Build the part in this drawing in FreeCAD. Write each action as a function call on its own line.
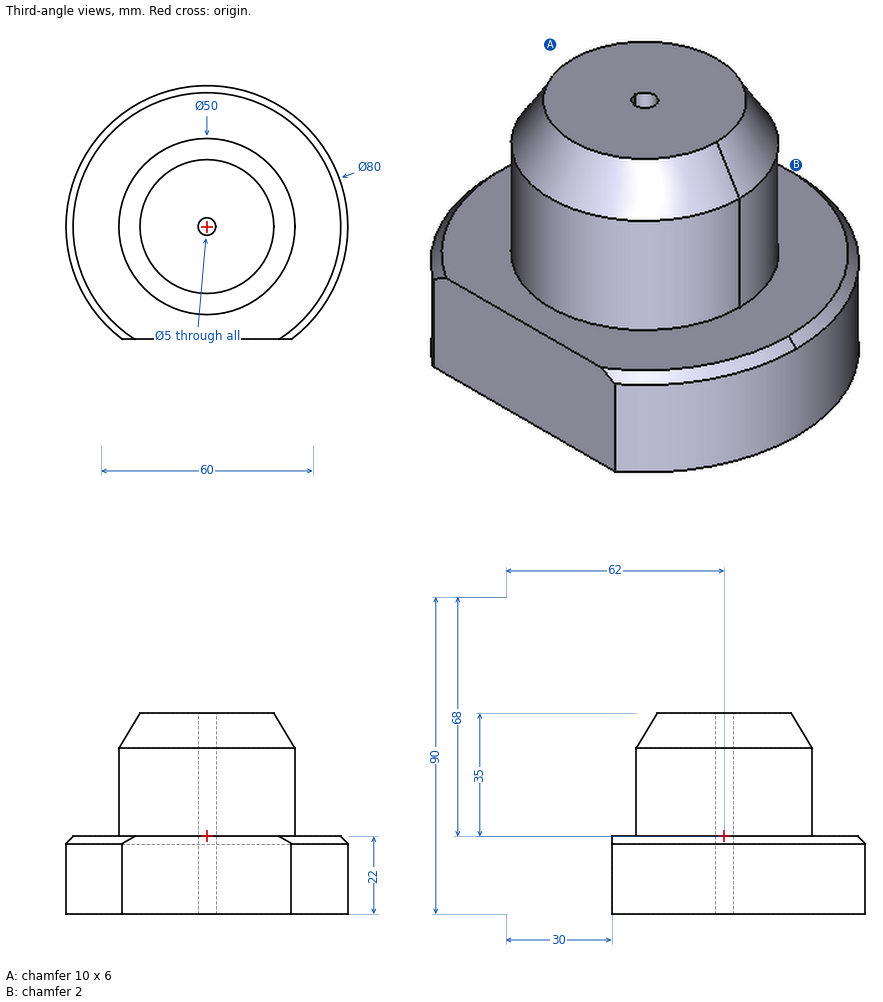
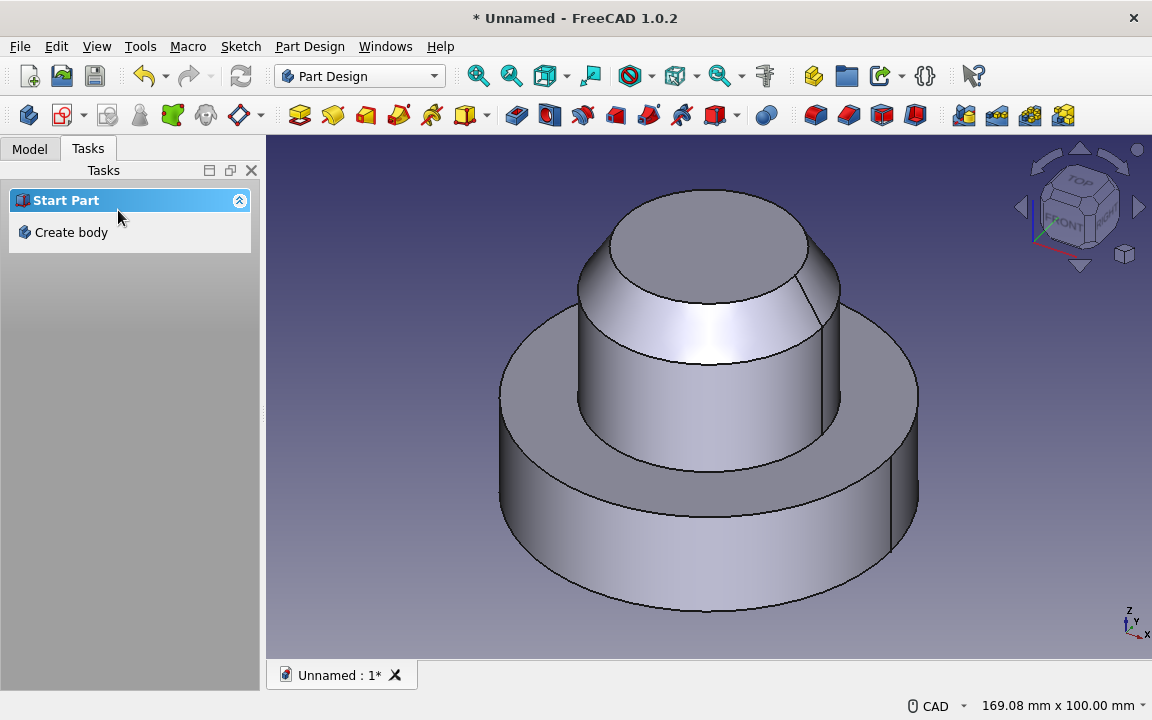
click(479, 76)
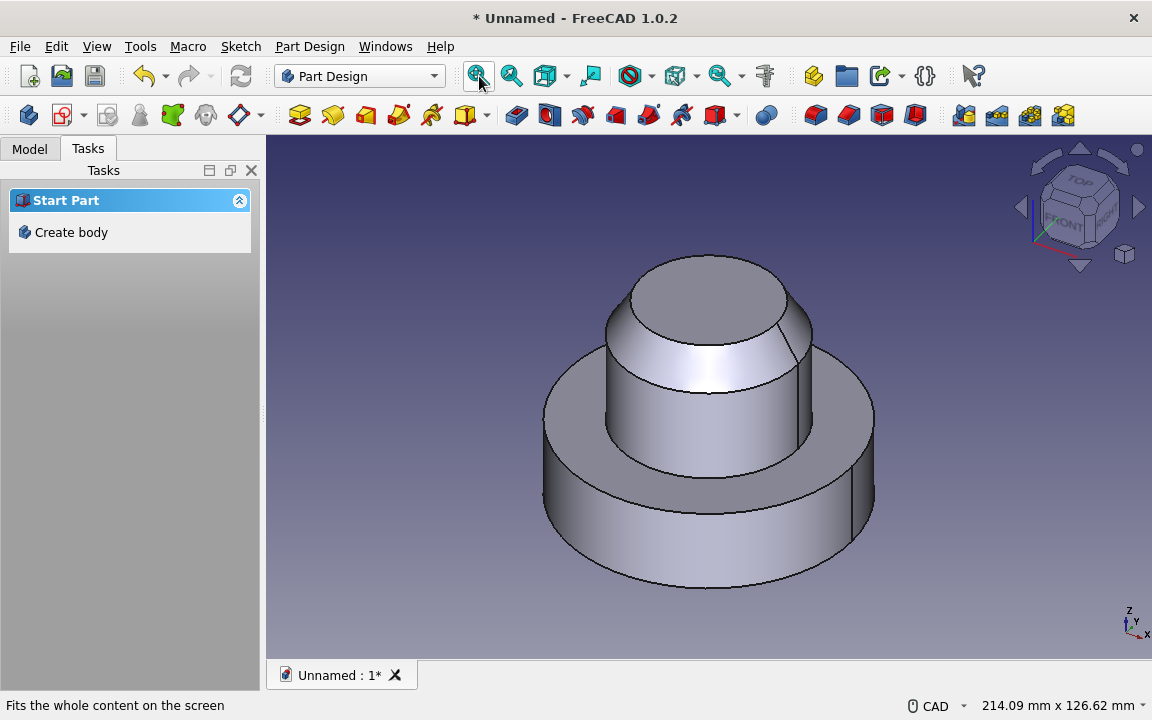
click(62, 116)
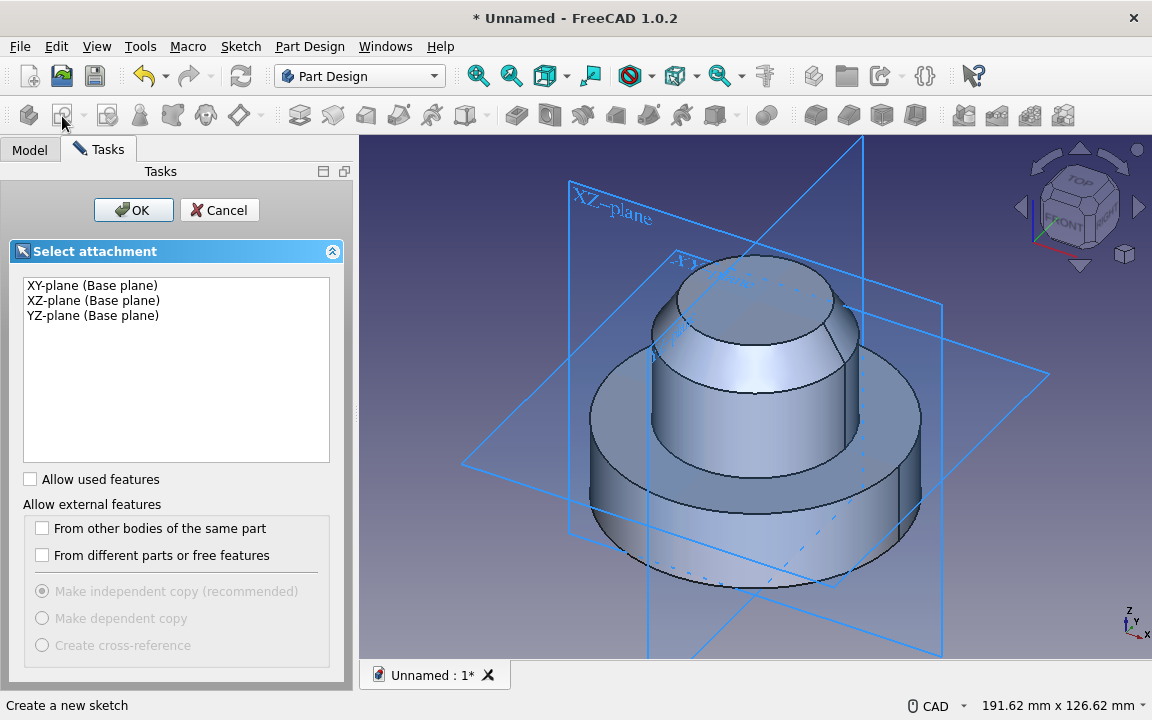
click(84, 316)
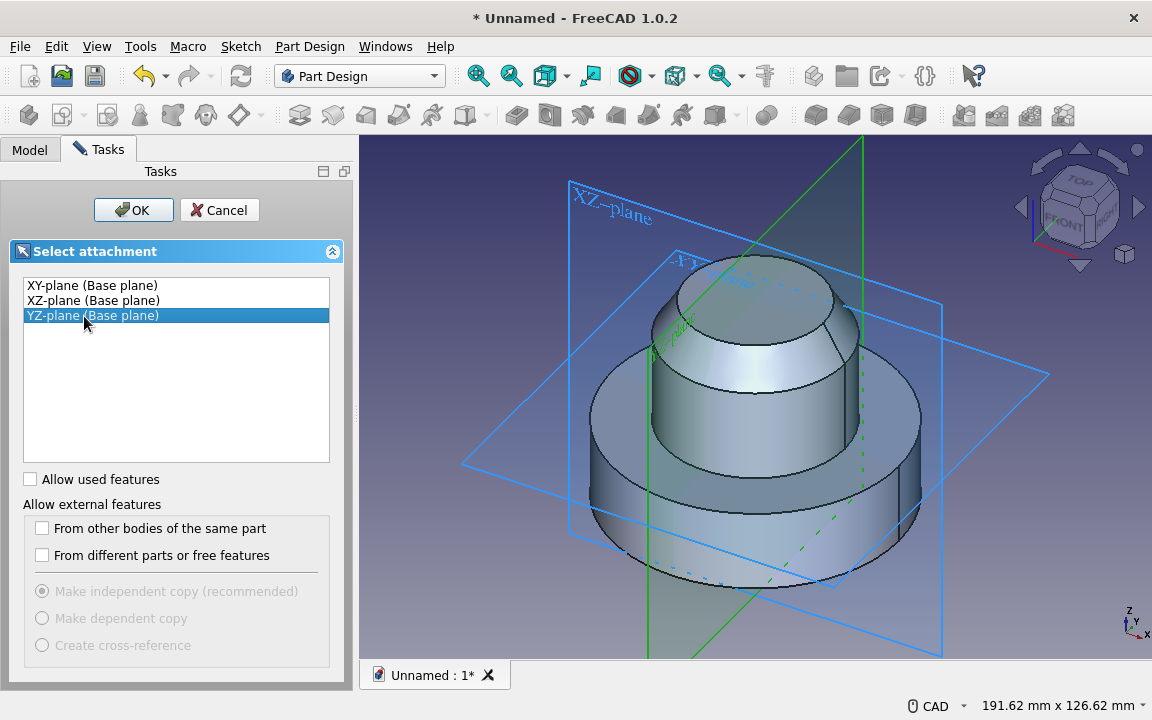
click(134, 210)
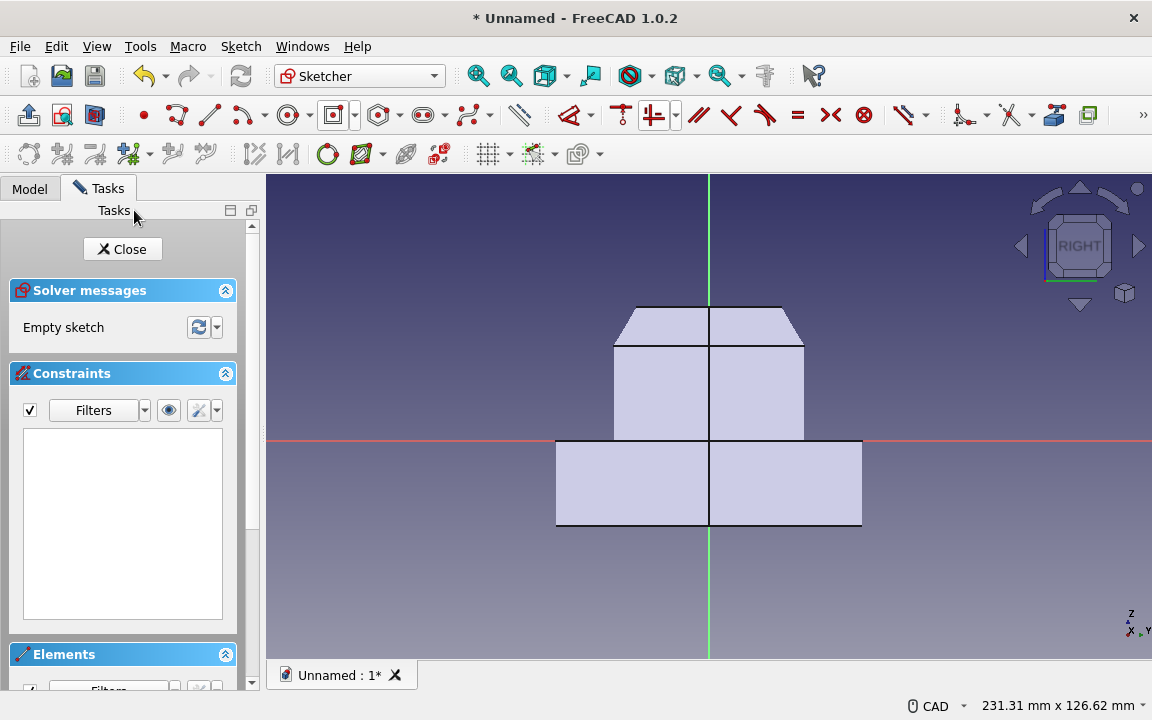
click(95, 116)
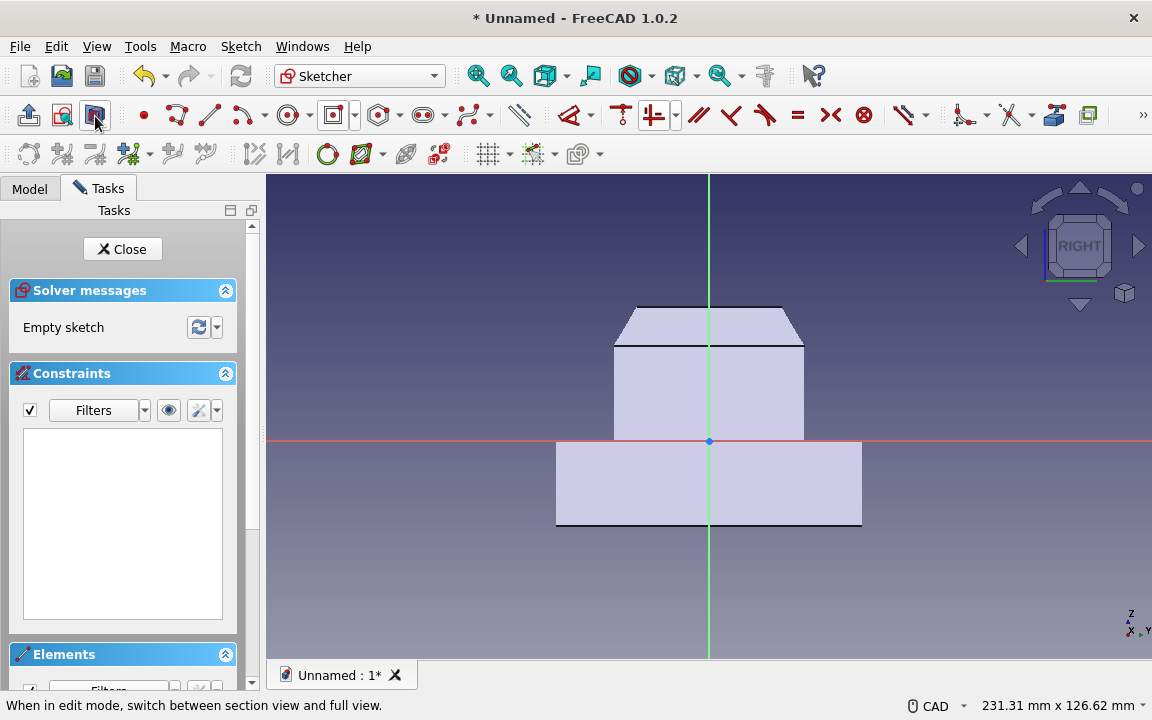
scroll(867, 631, down, 1)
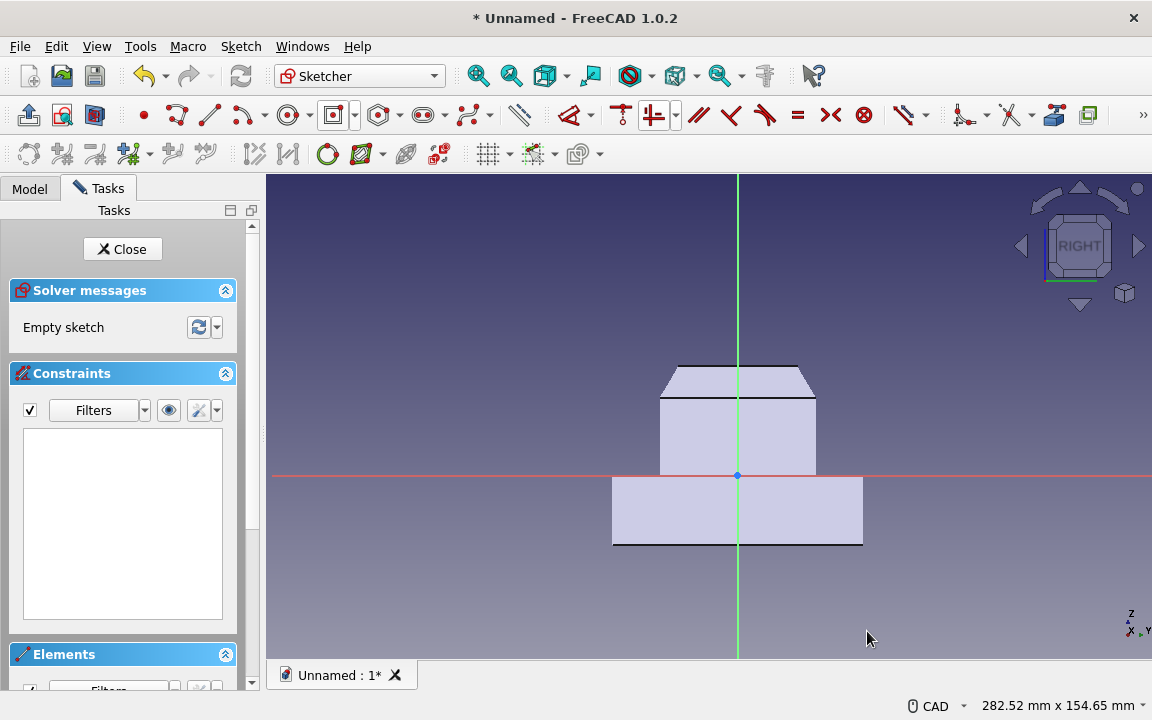
click(354, 116)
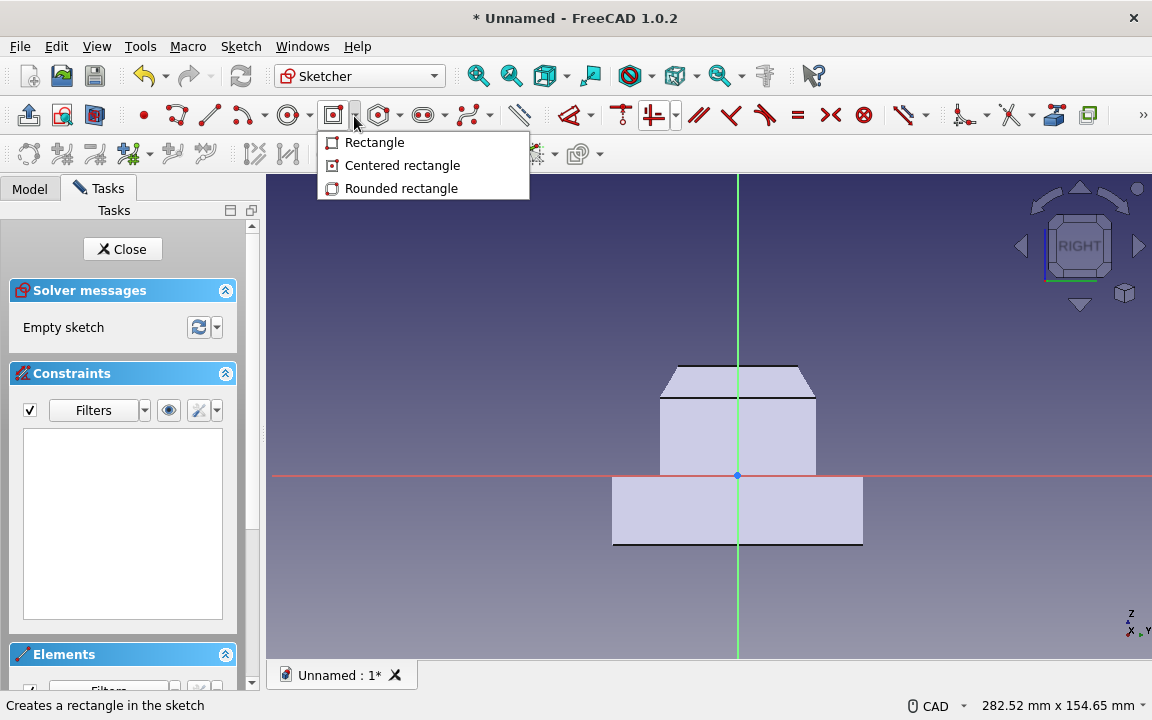
click(424, 142)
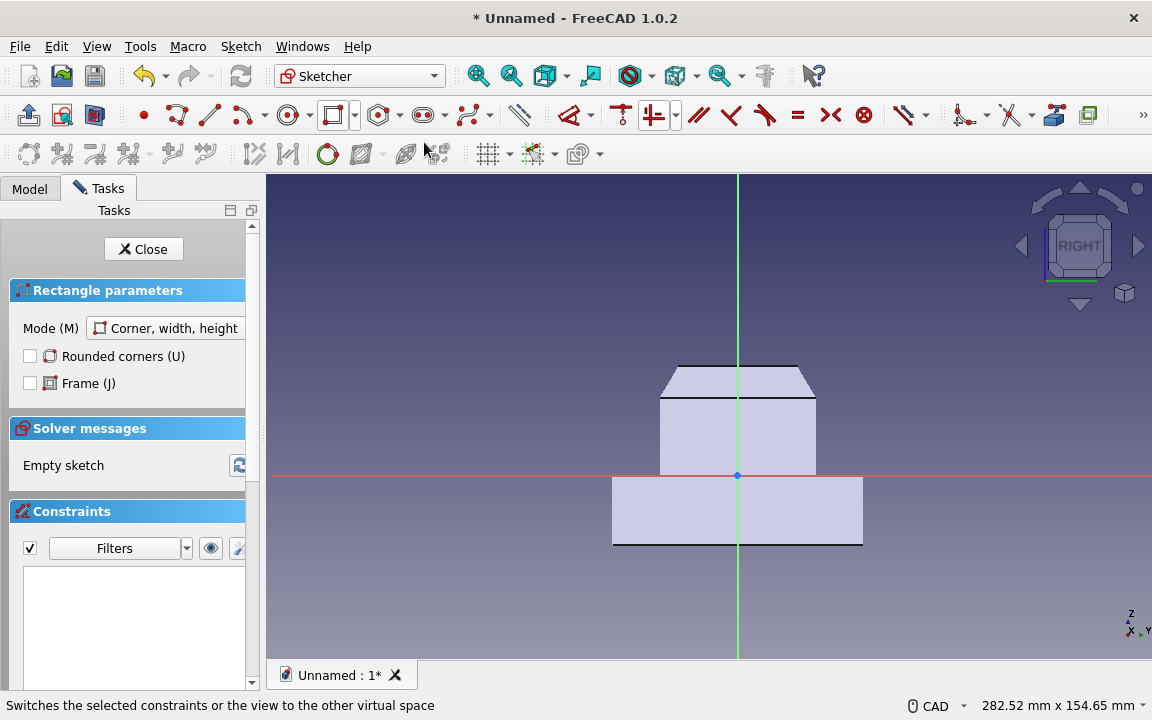
click(543, 263)
click(637, 545)
key(Escape)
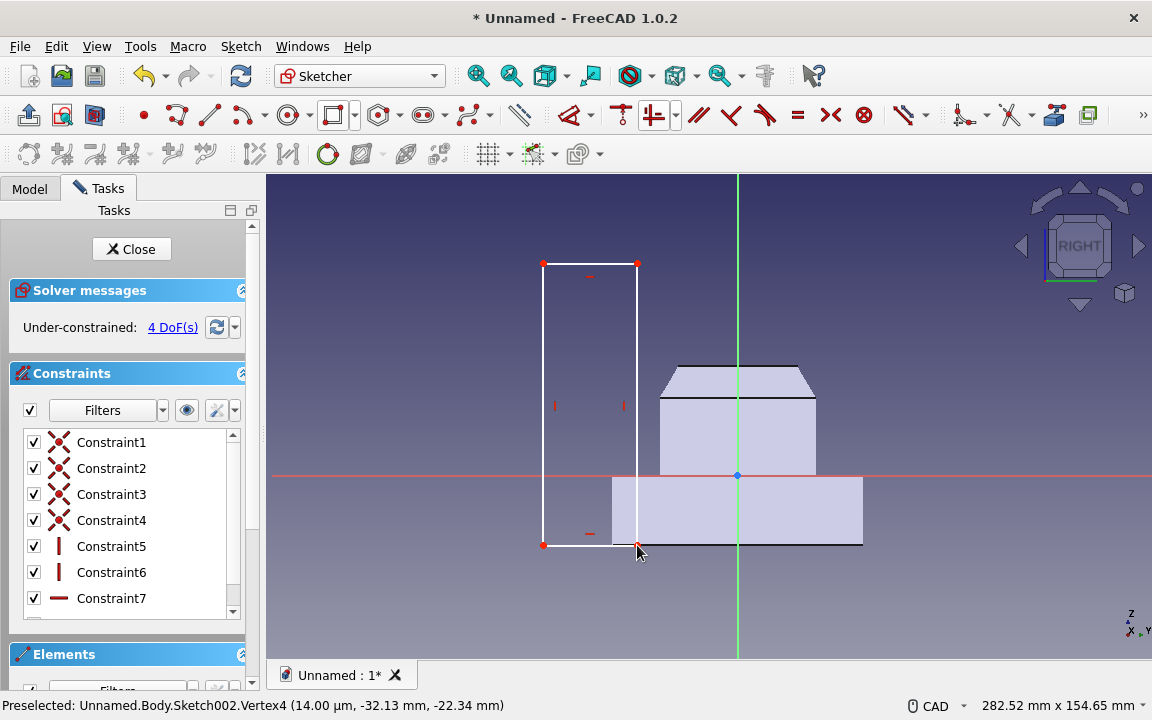
key(d)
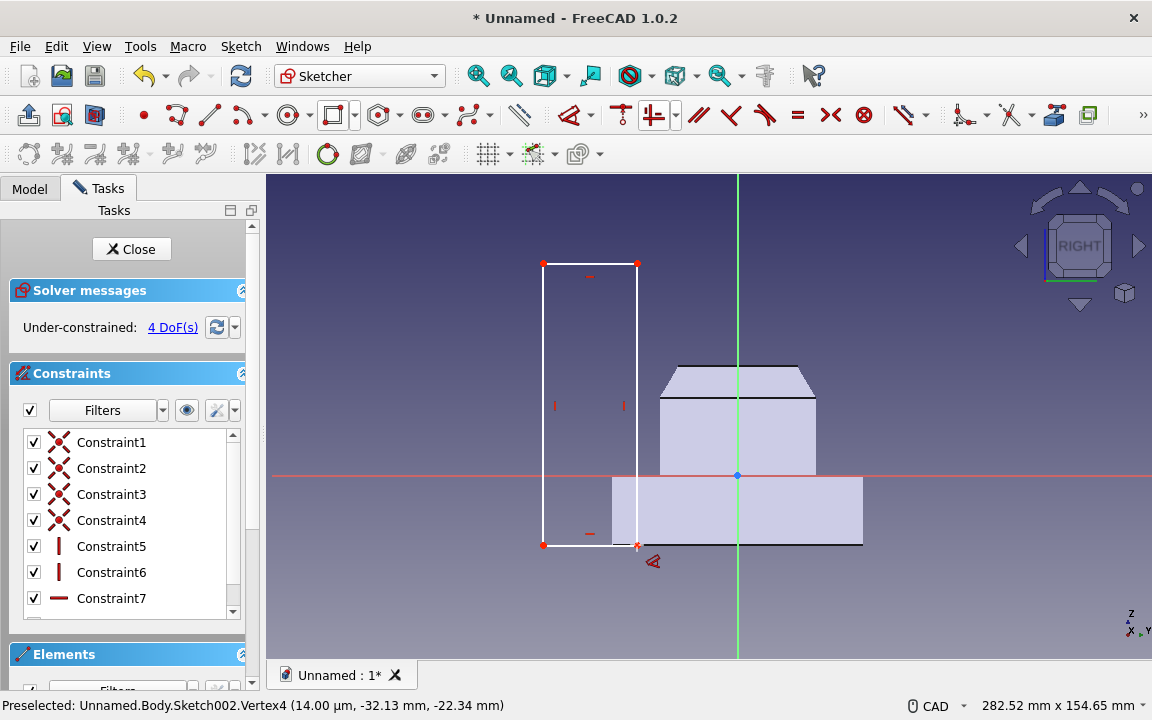
click(543, 349)
click(509, 405)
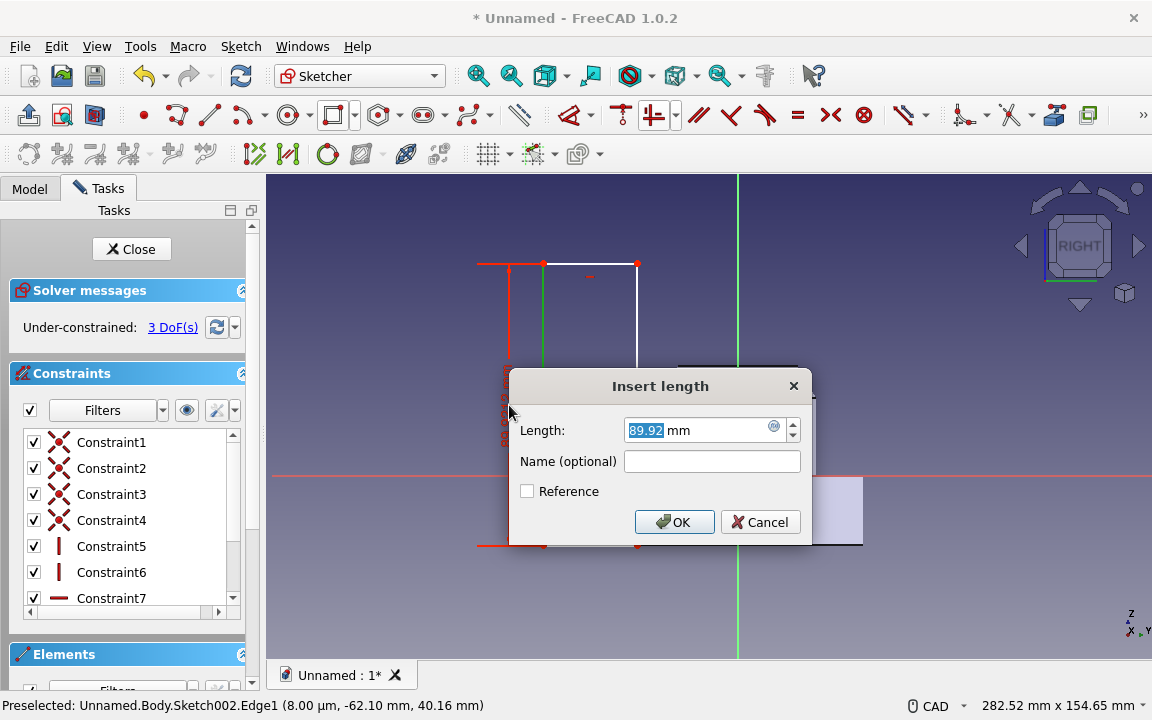
text(90)
key(Return)